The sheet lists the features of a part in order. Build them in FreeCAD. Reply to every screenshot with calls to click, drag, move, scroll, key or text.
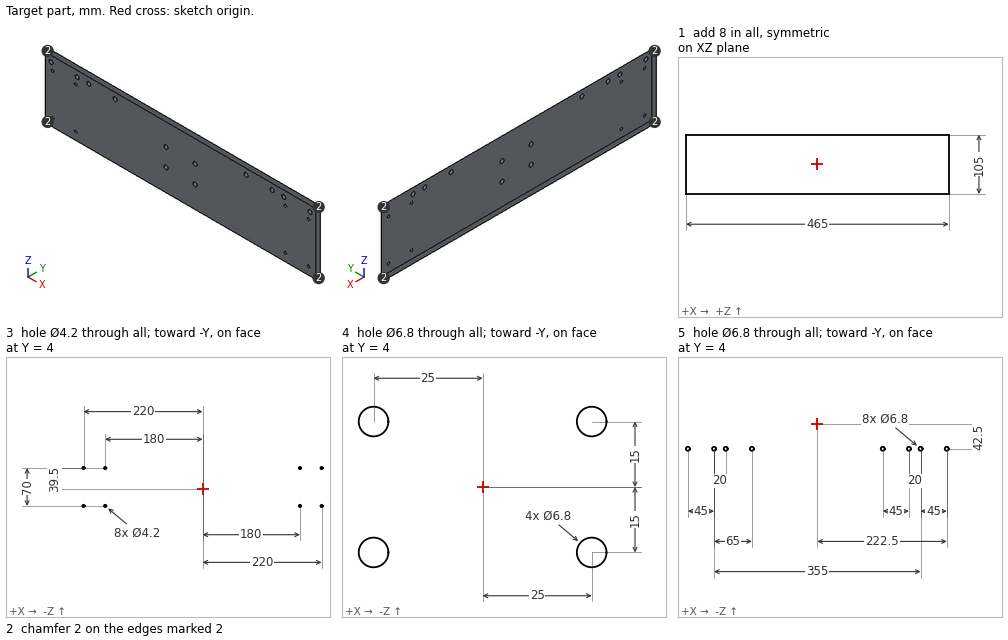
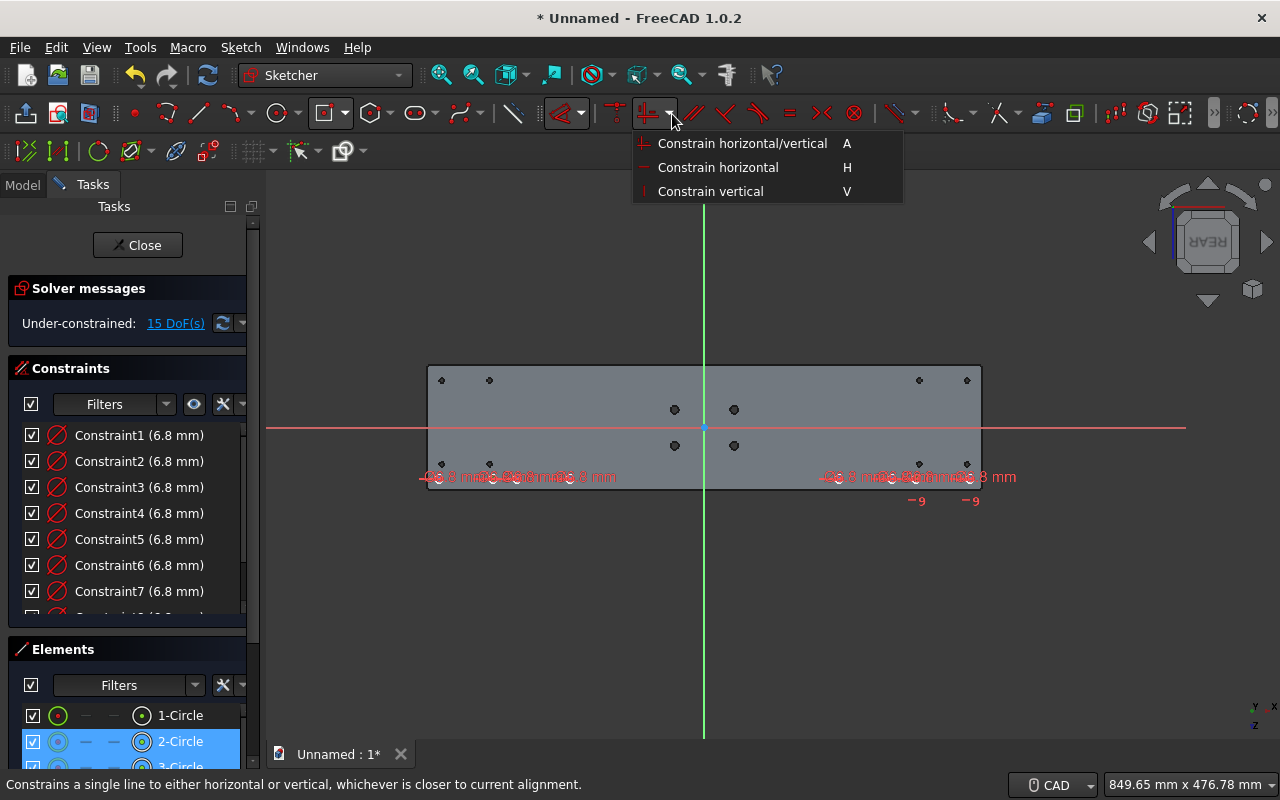
click(768, 167)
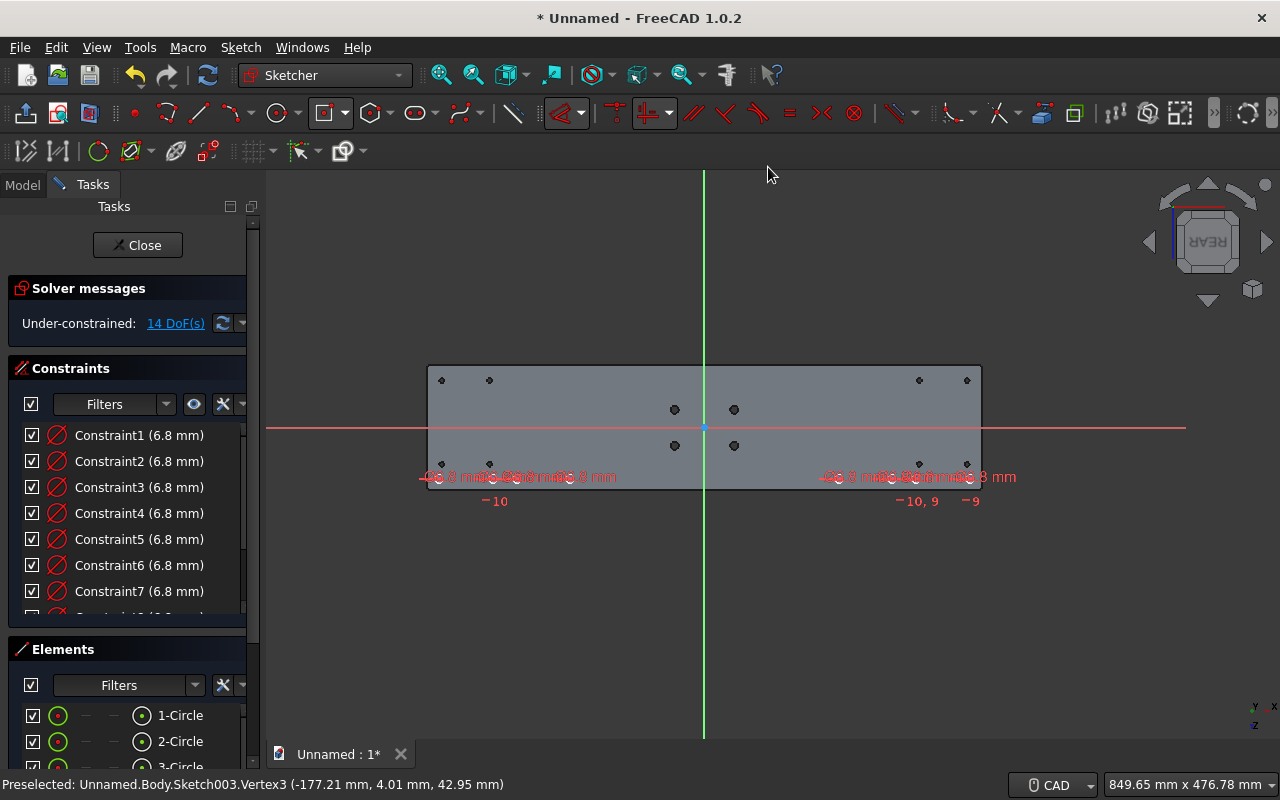
click(493, 479)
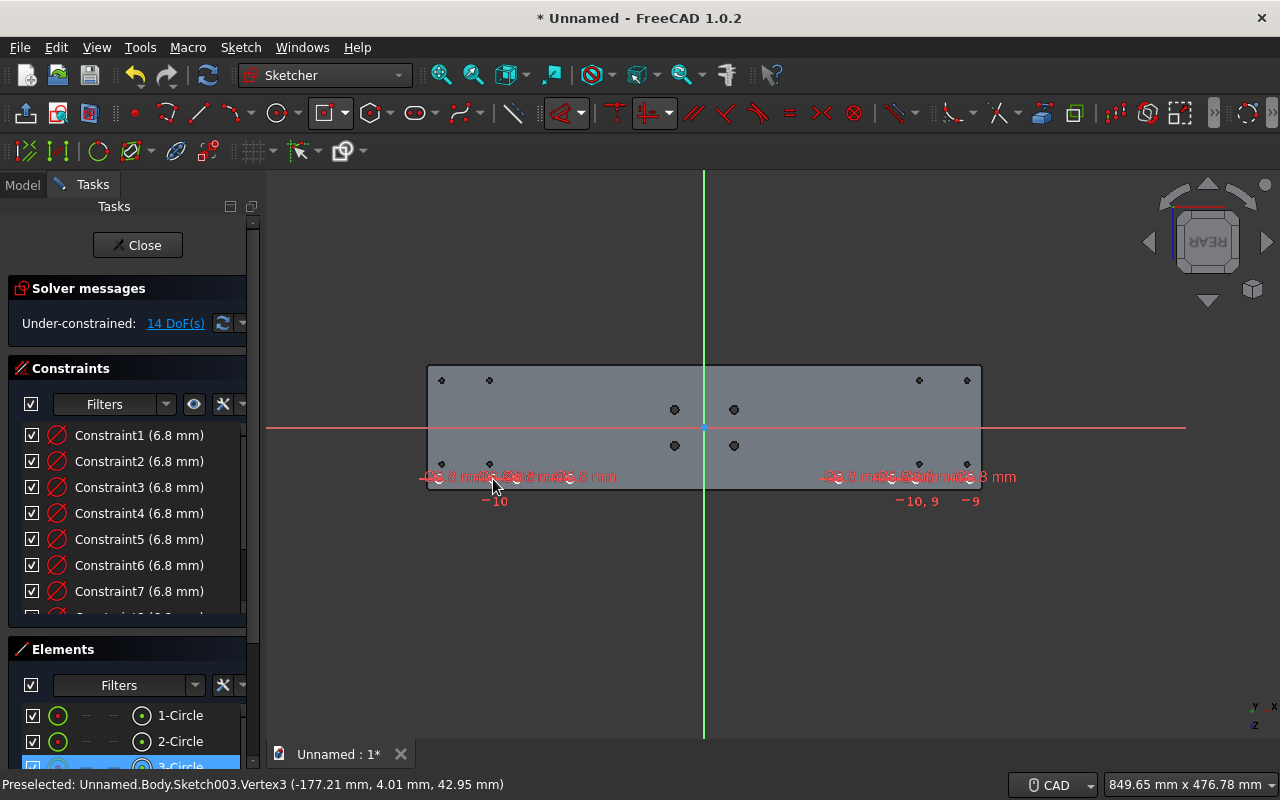
click(439, 479)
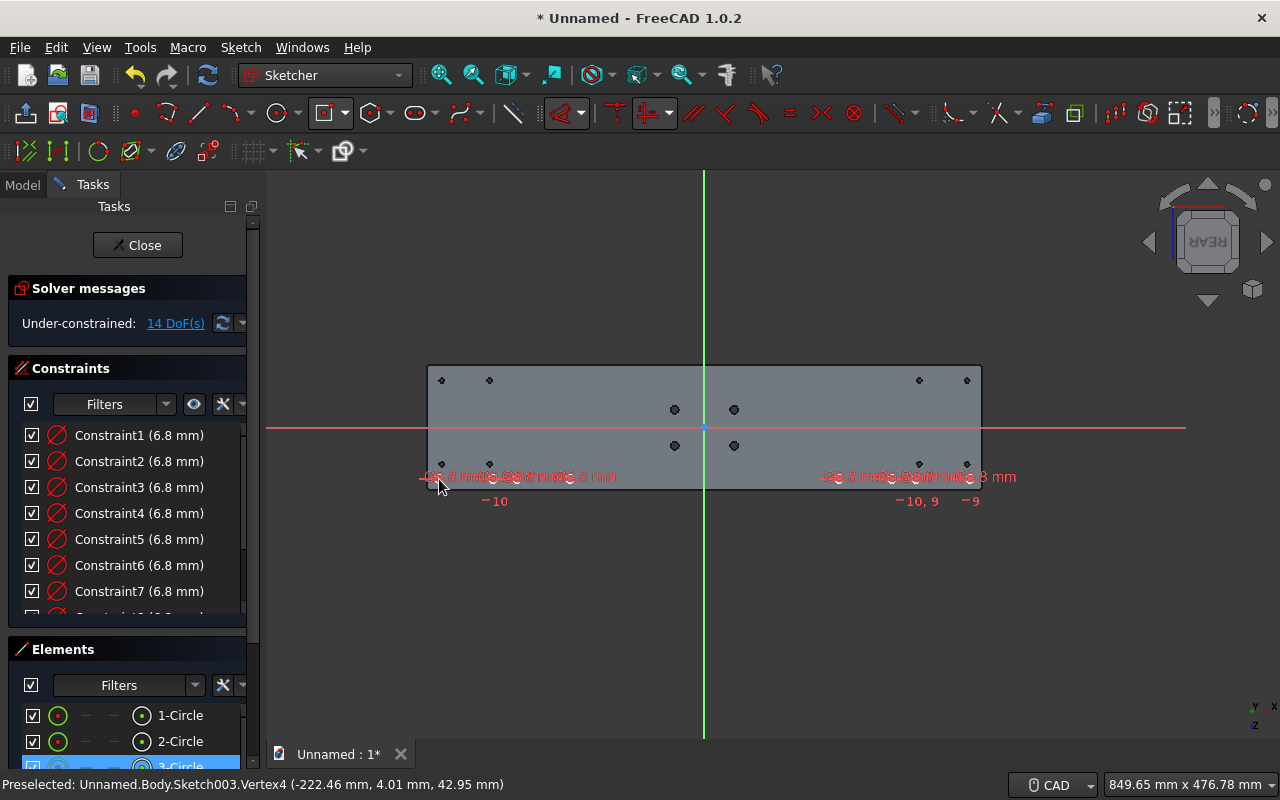
key(h)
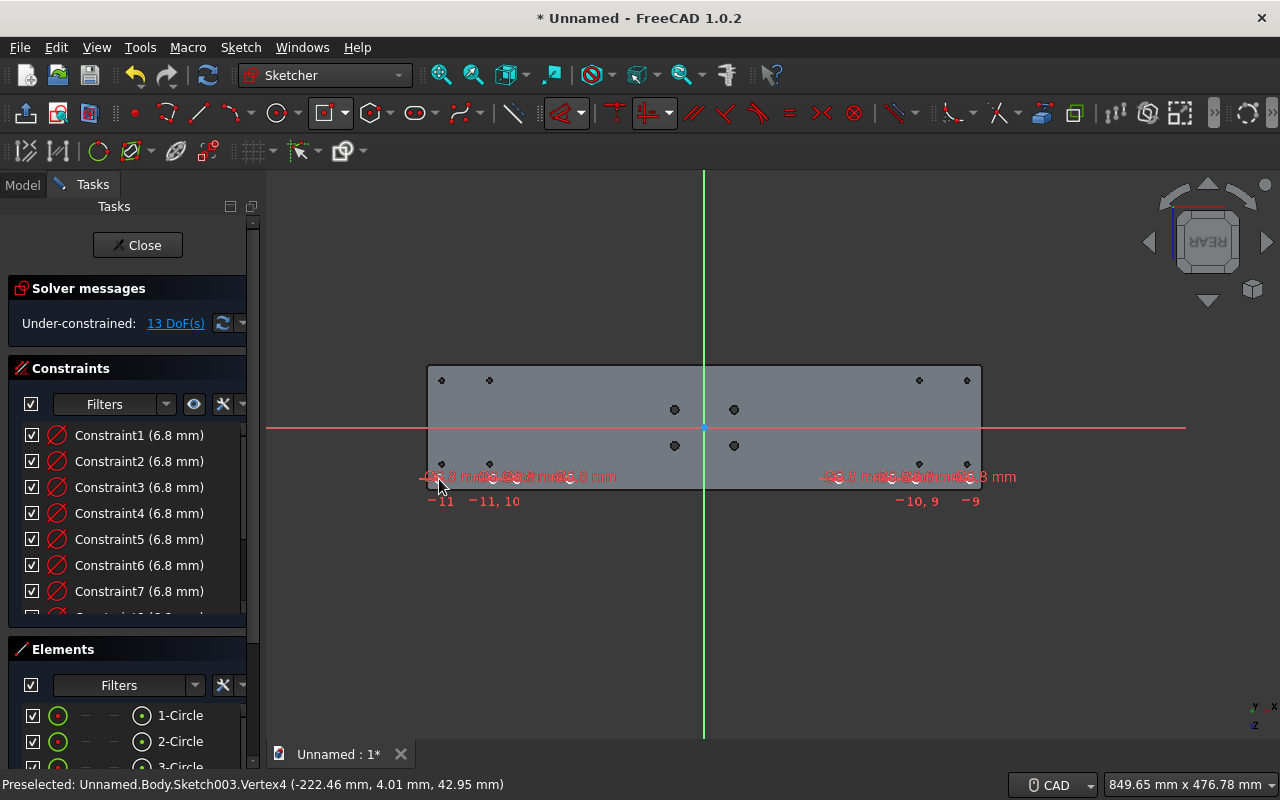
click(916, 479)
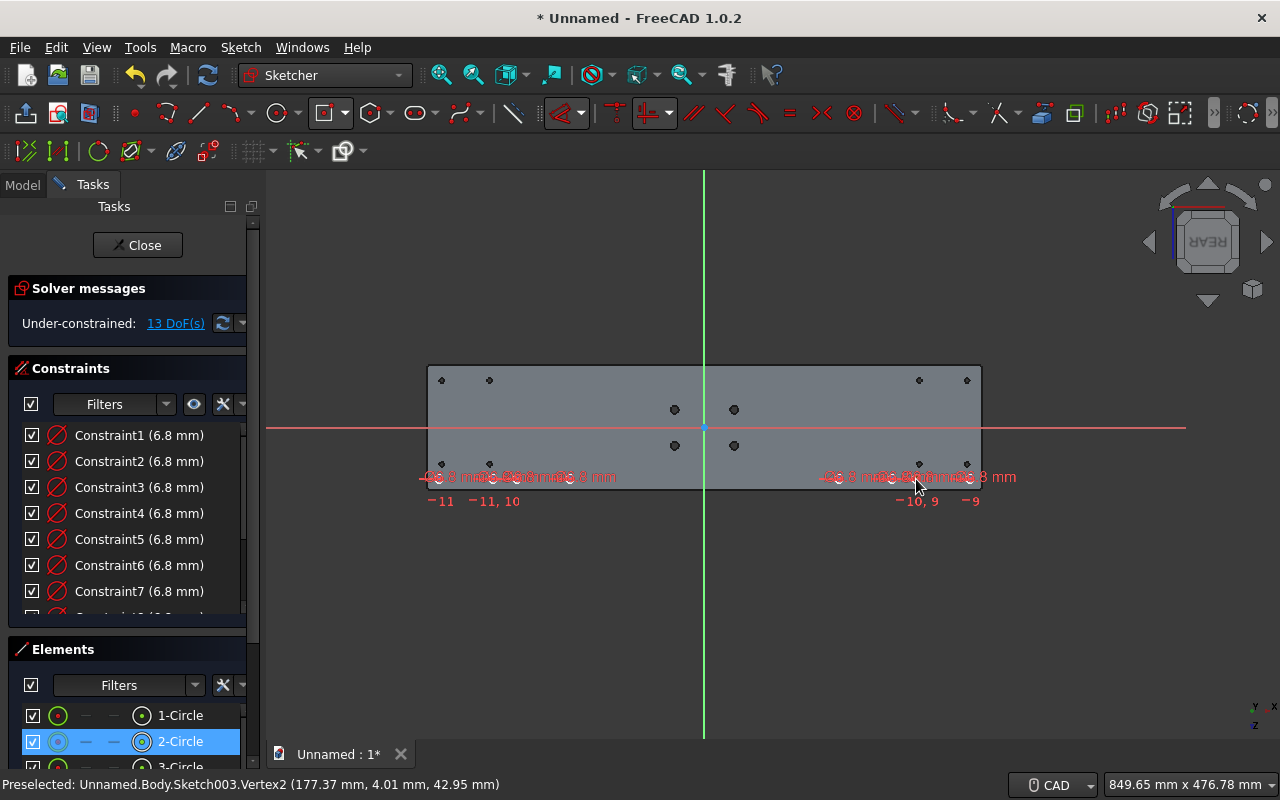
click(892, 479)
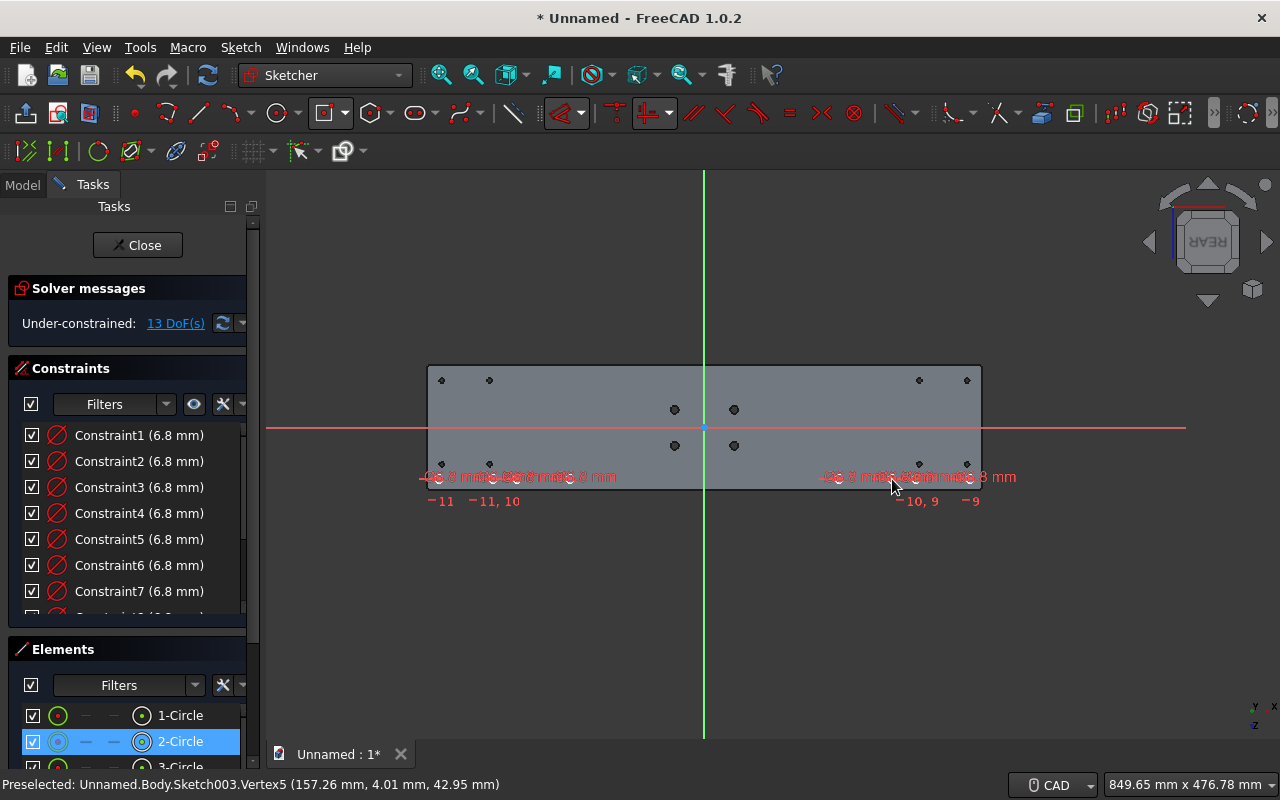
key(h)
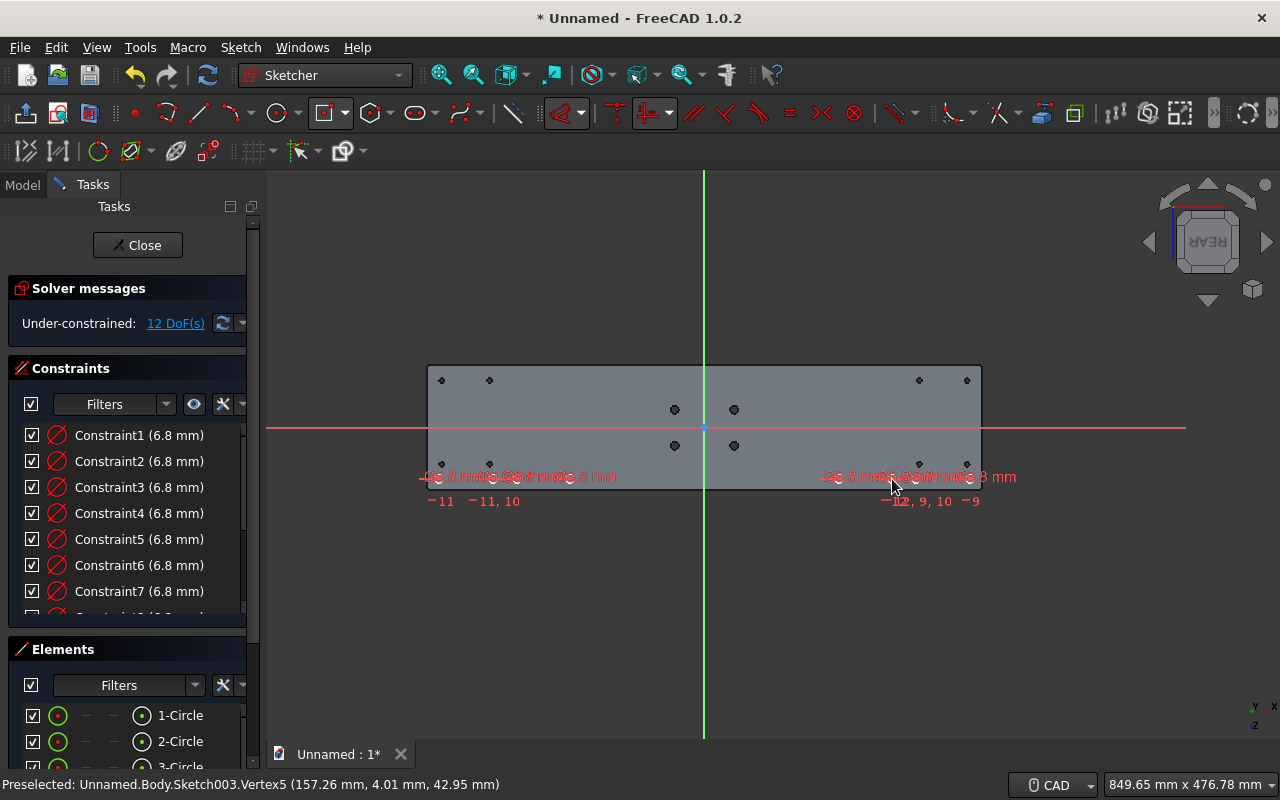
click(892, 479)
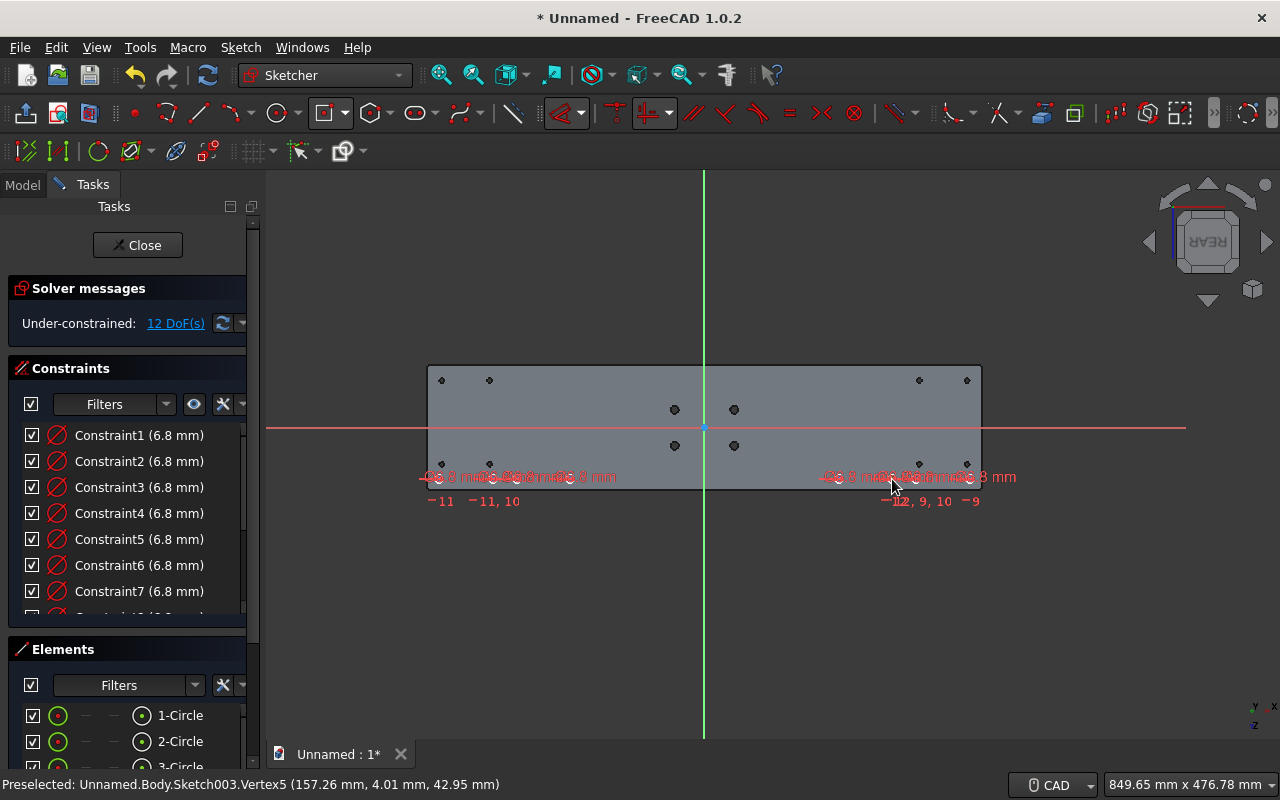
click(839, 479)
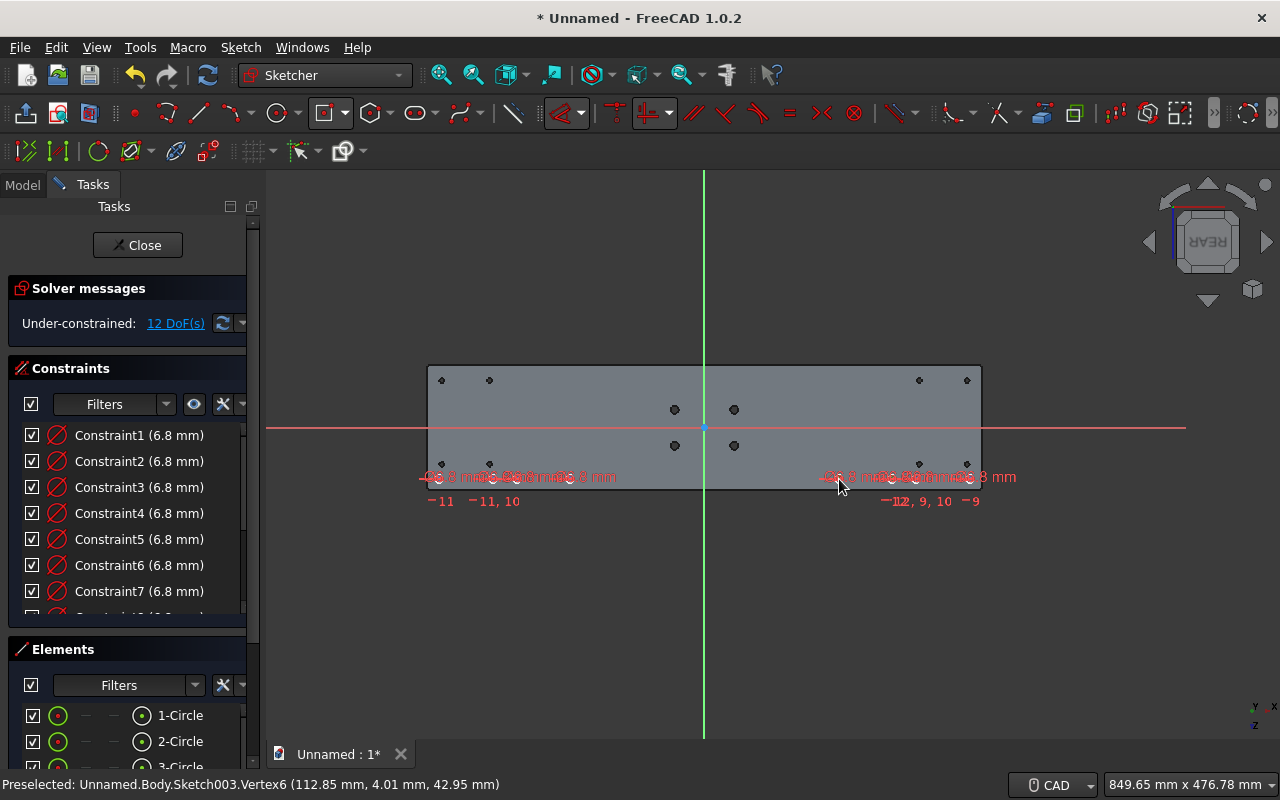
click(672, 114)